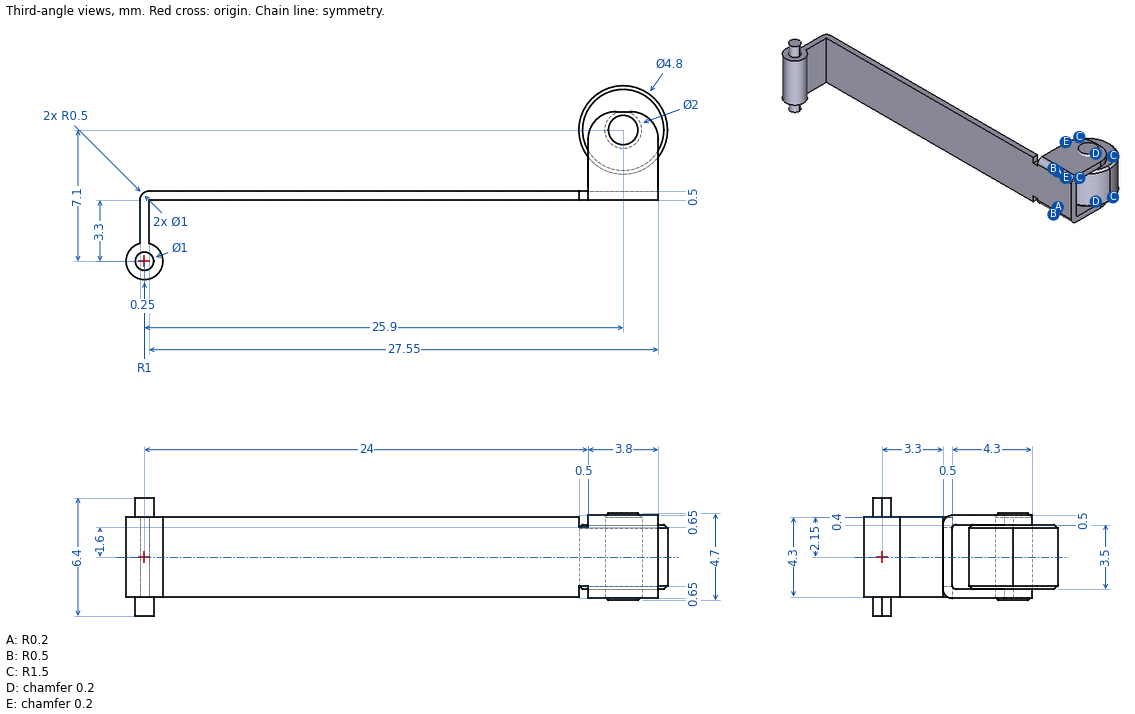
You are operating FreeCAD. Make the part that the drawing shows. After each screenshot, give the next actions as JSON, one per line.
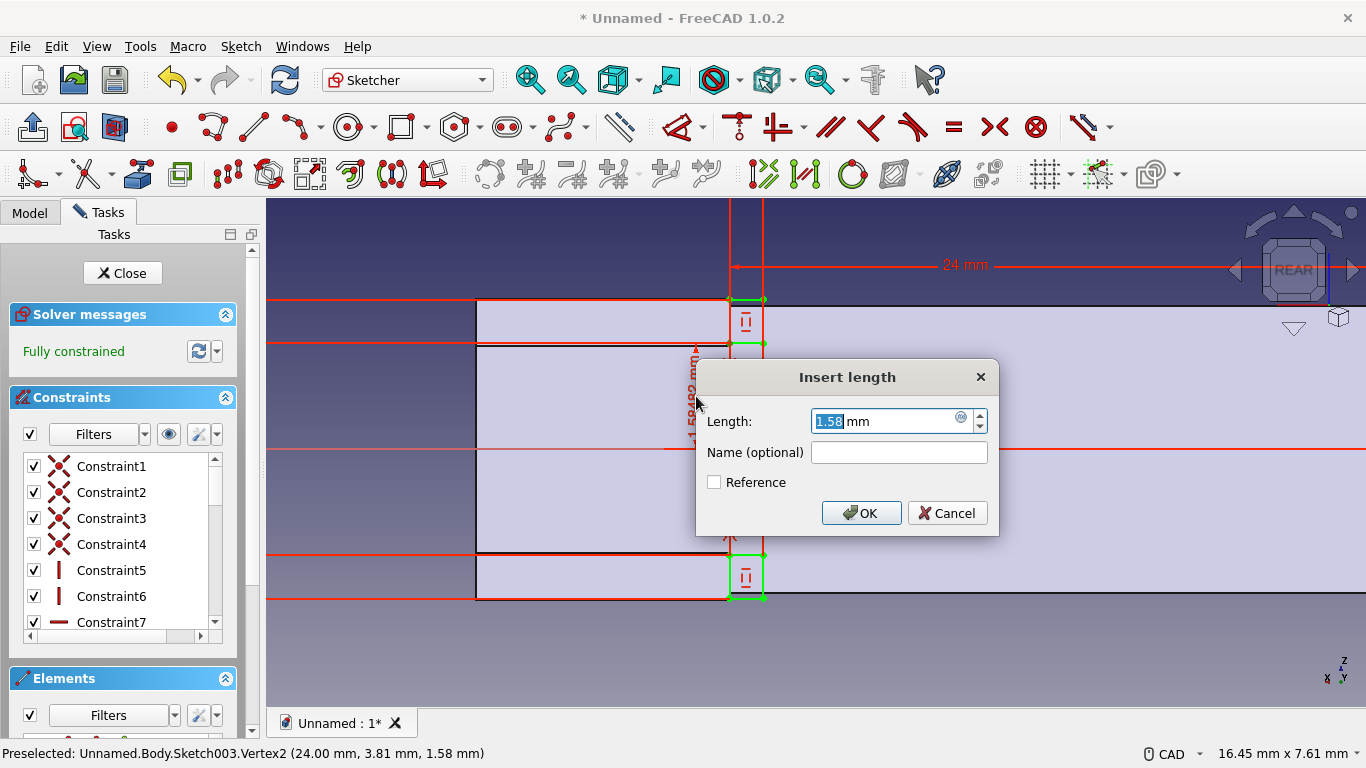
{"action": "type", "text": "1.6"}
{"action": "key", "text": "Return"}
{"action": "key", "text": "Escape"}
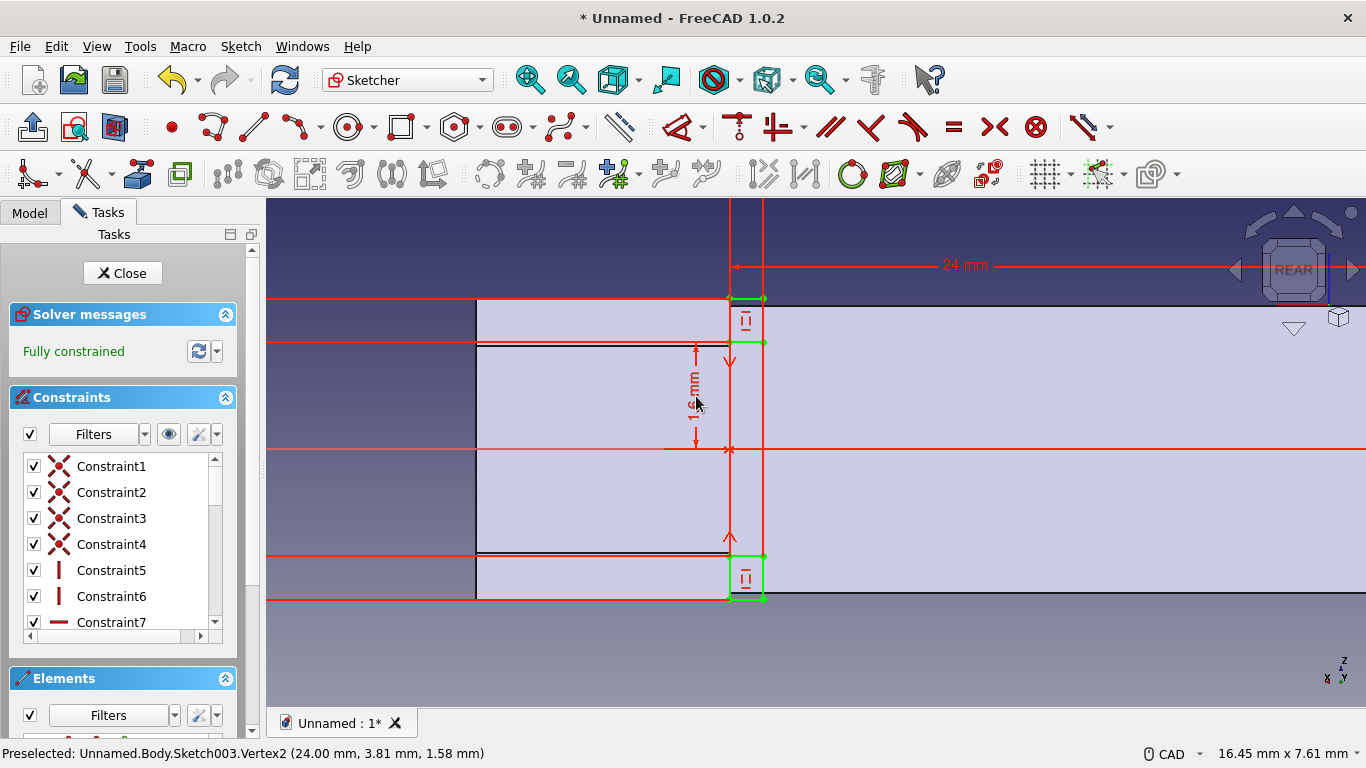
{"action": "left_click", "coordinate": [123, 273]}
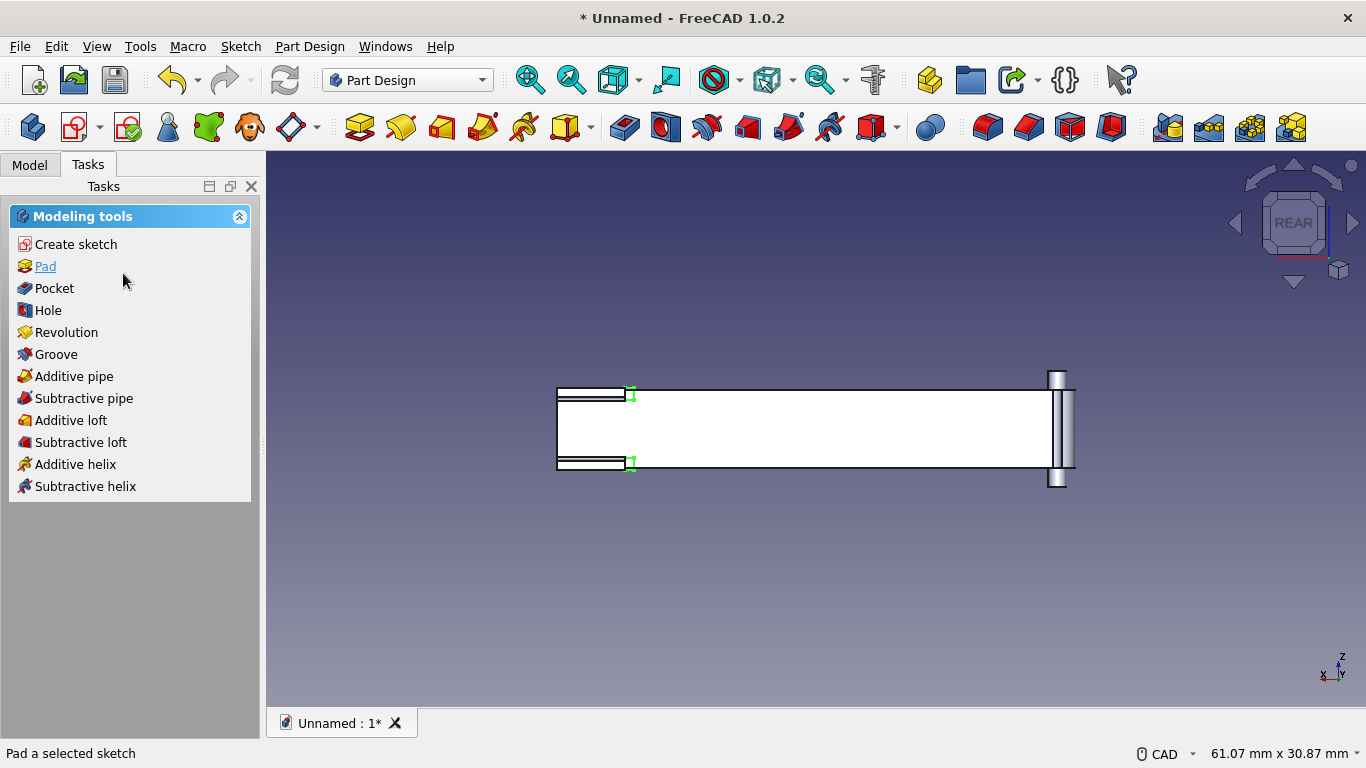
{"action": "left_click", "coordinate": [625, 128]}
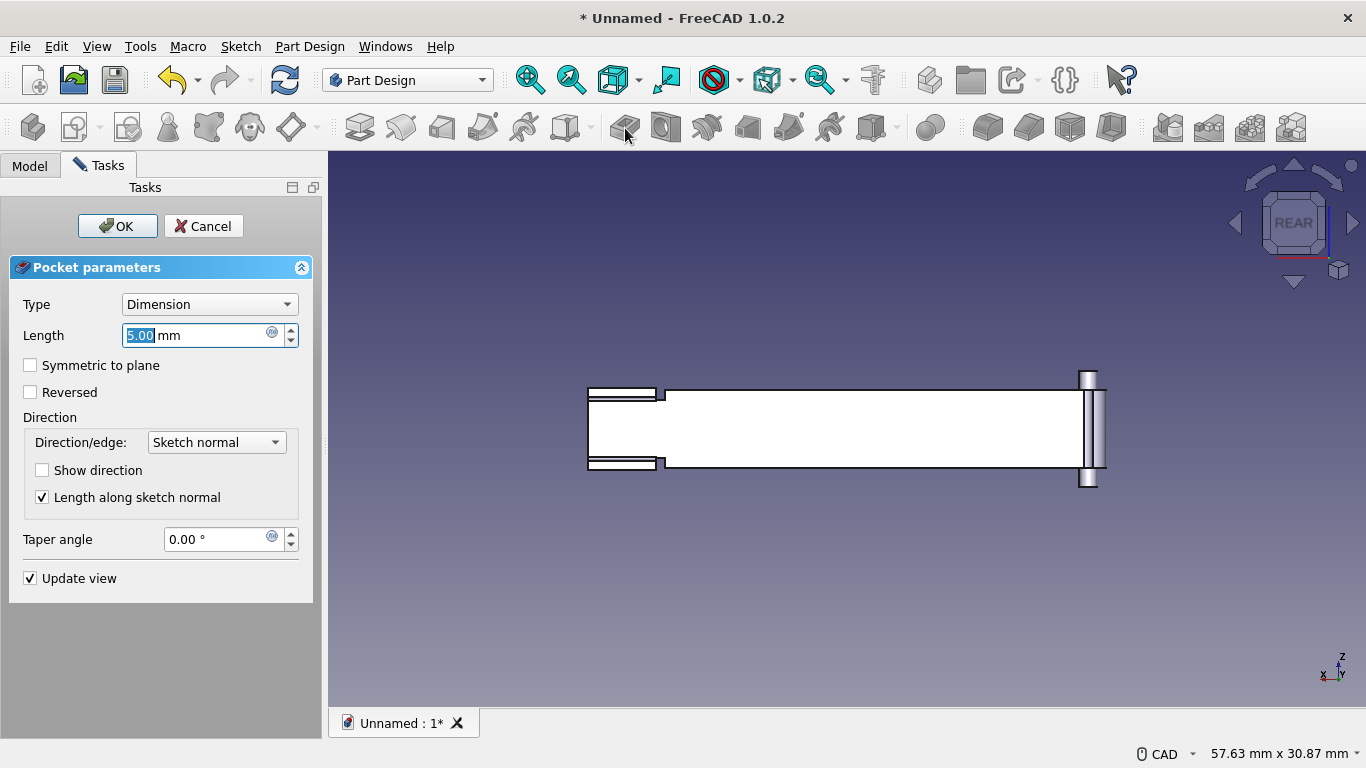
{"action": "left_click", "coordinate": [210, 304]}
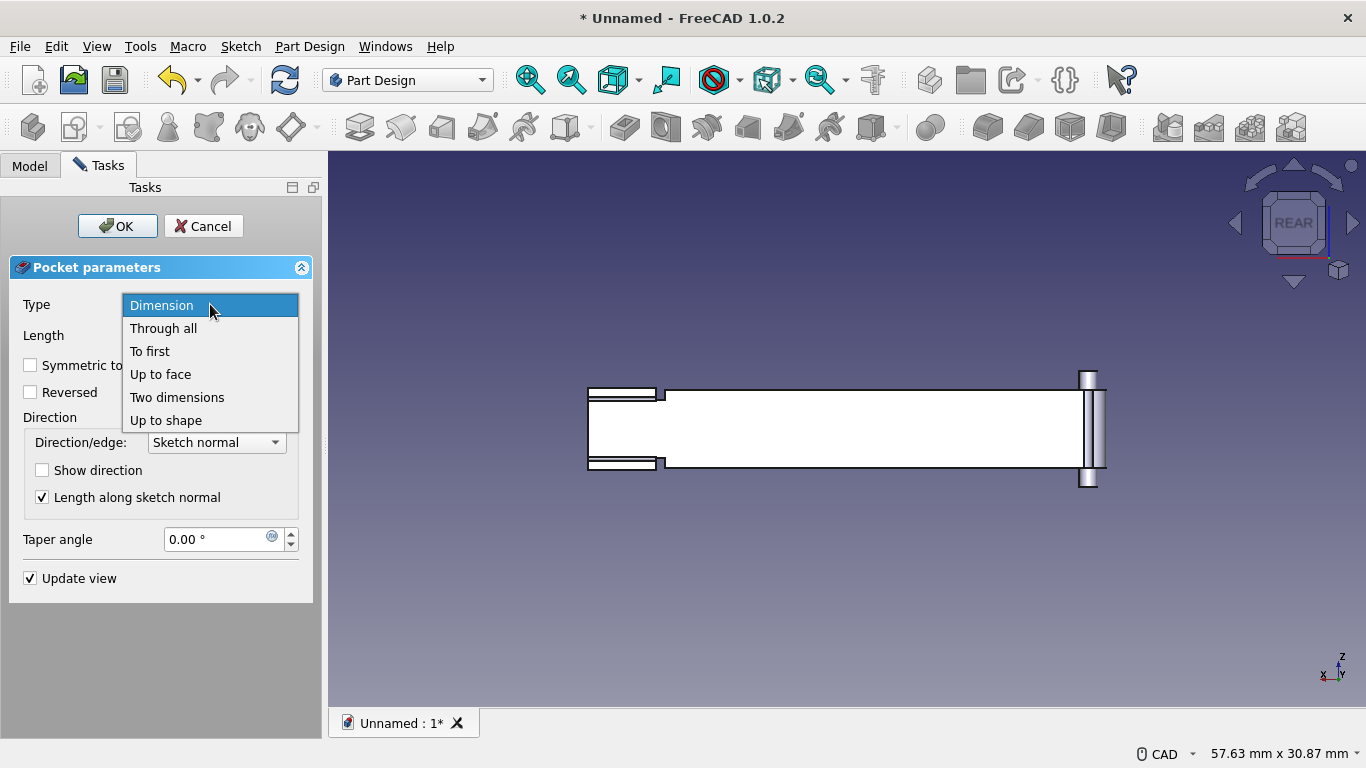
{"action": "left_click", "coordinate": [208, 328]}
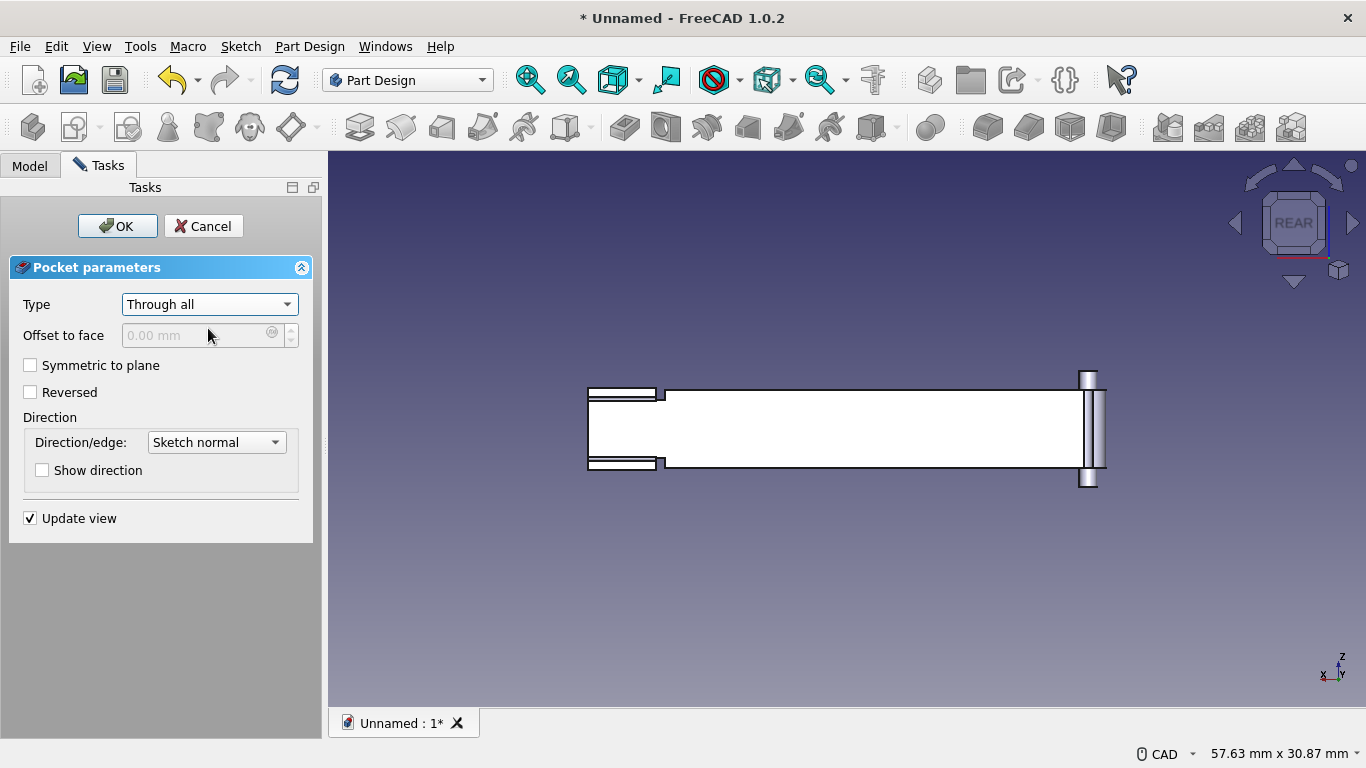
{"action": "left_click", "coordinate": [118, 226]}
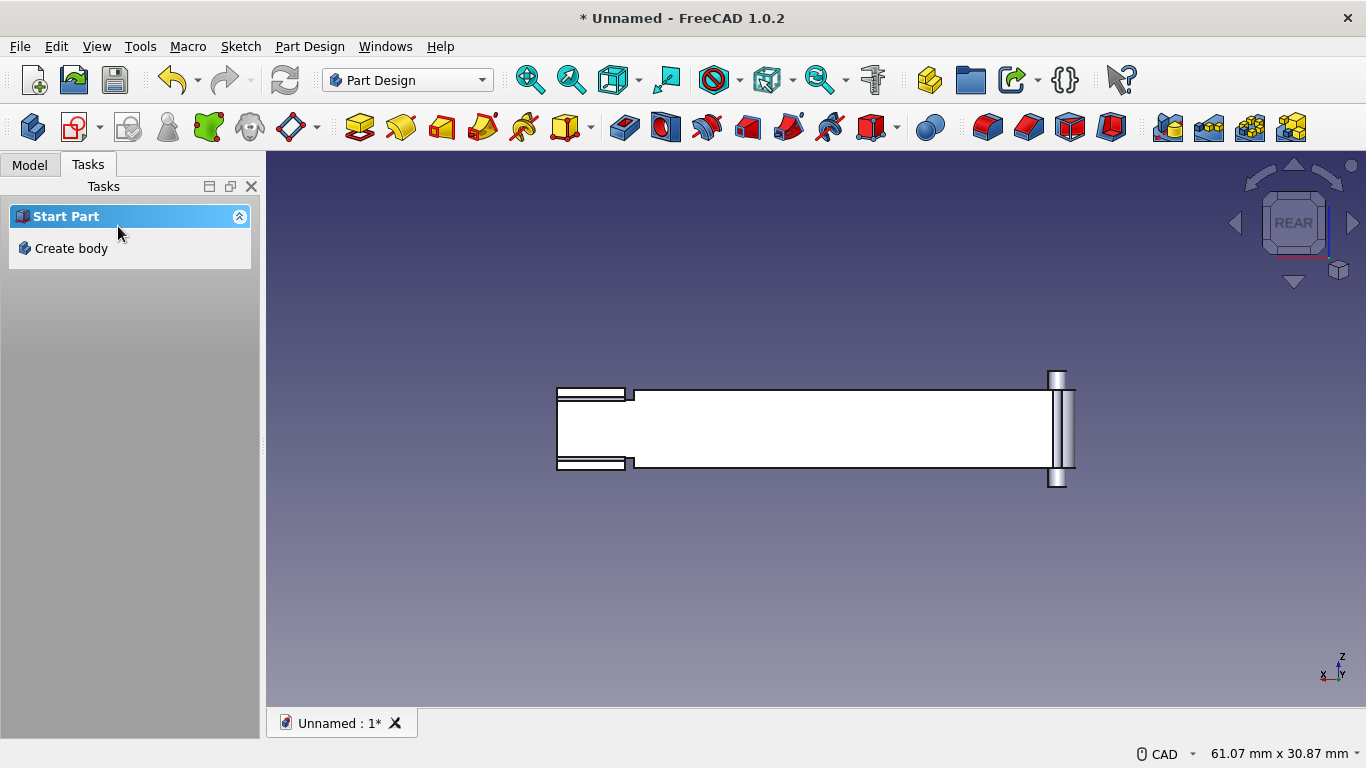
{"action": "key", "text": "0"}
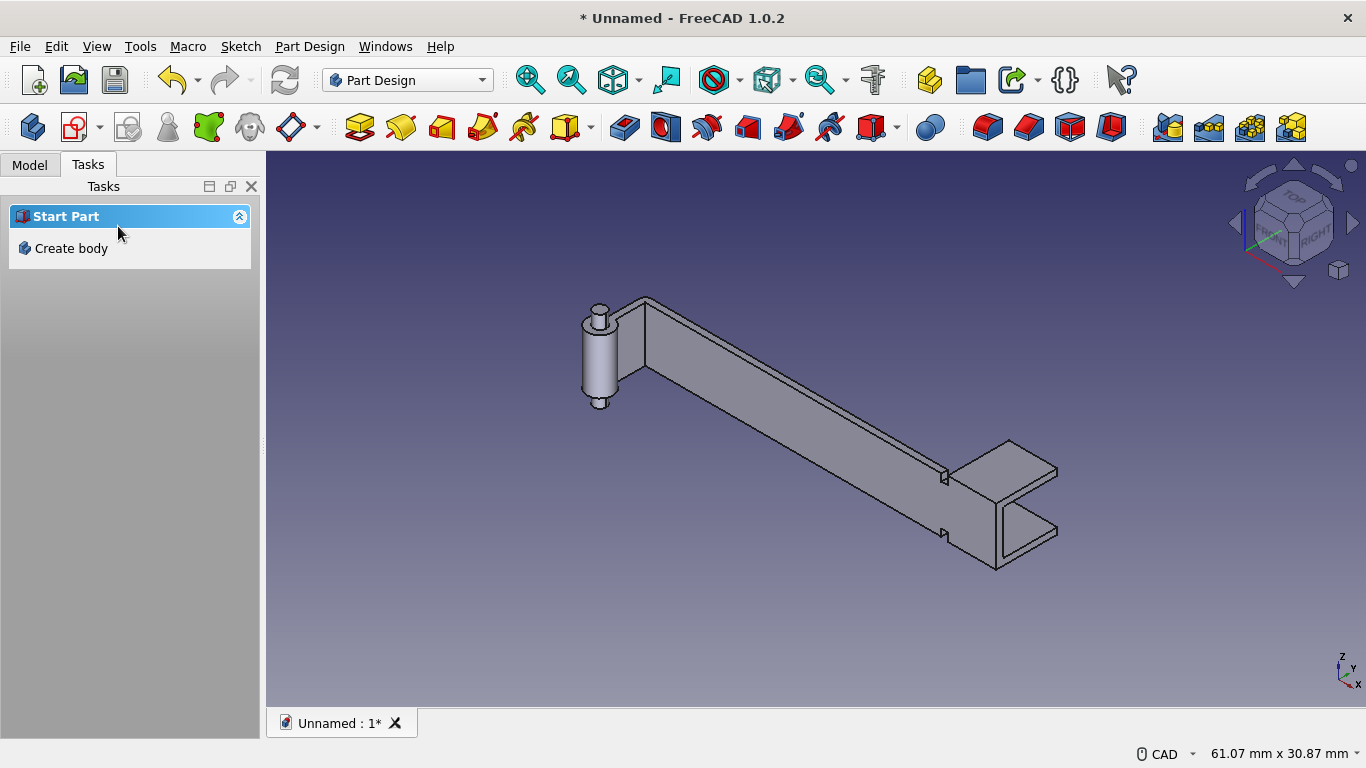
{"action": "left_click", "coordinate": [972, 489]}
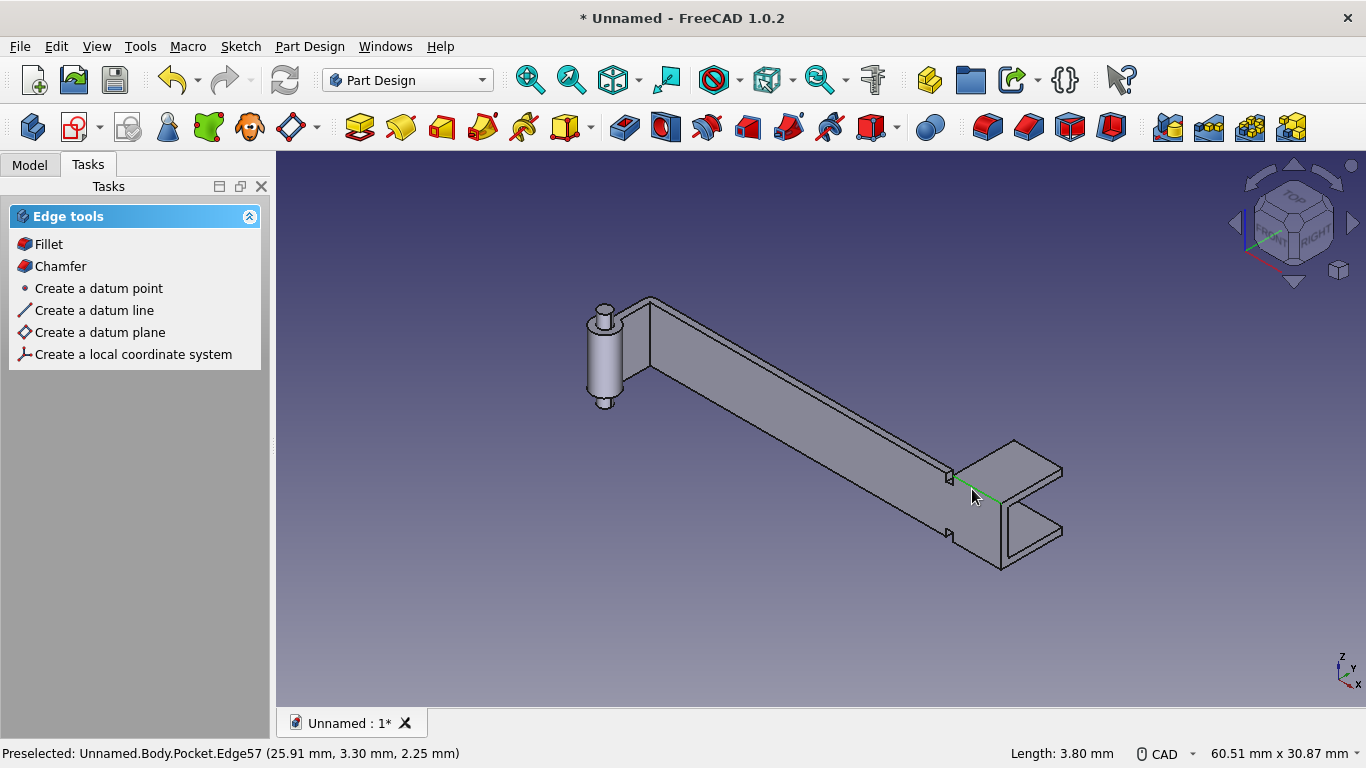
{"action": "key", "text": "2"}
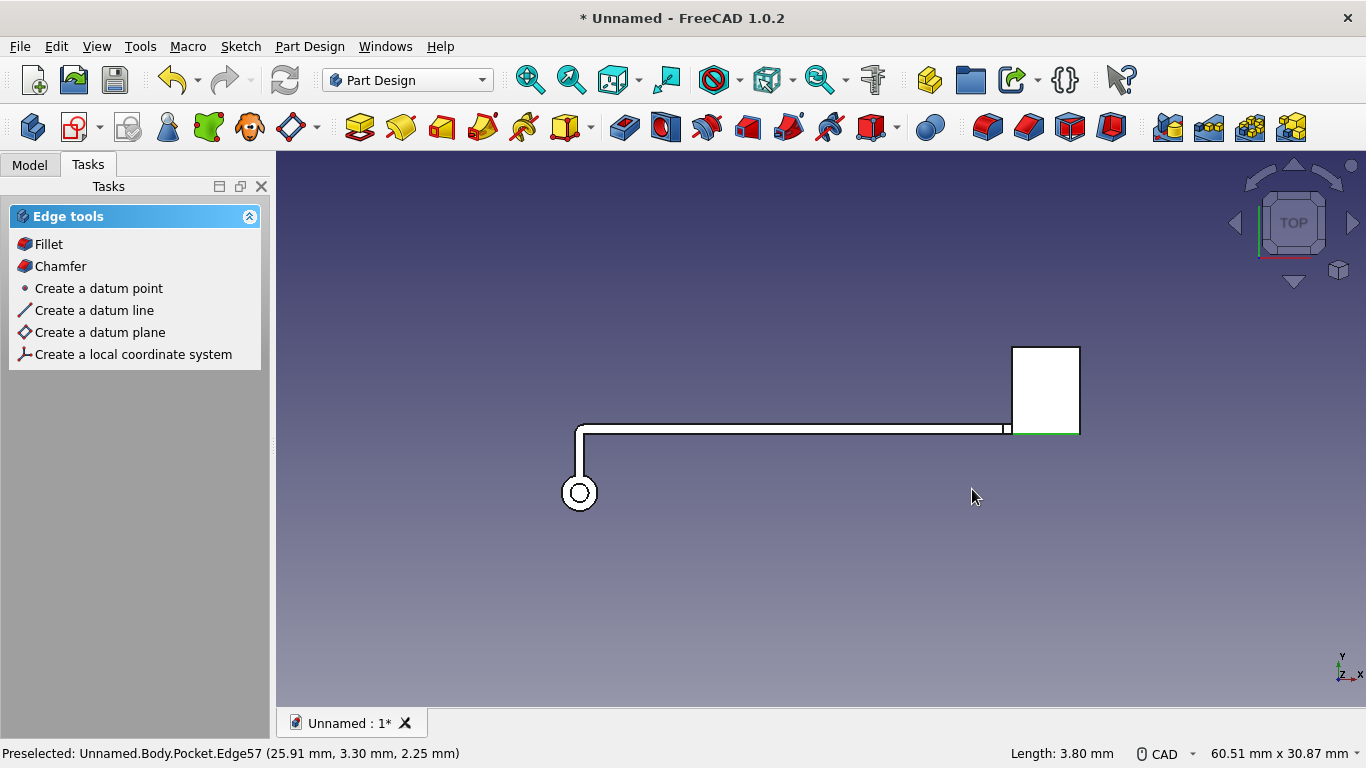
{"action": "key", "text": "1"}